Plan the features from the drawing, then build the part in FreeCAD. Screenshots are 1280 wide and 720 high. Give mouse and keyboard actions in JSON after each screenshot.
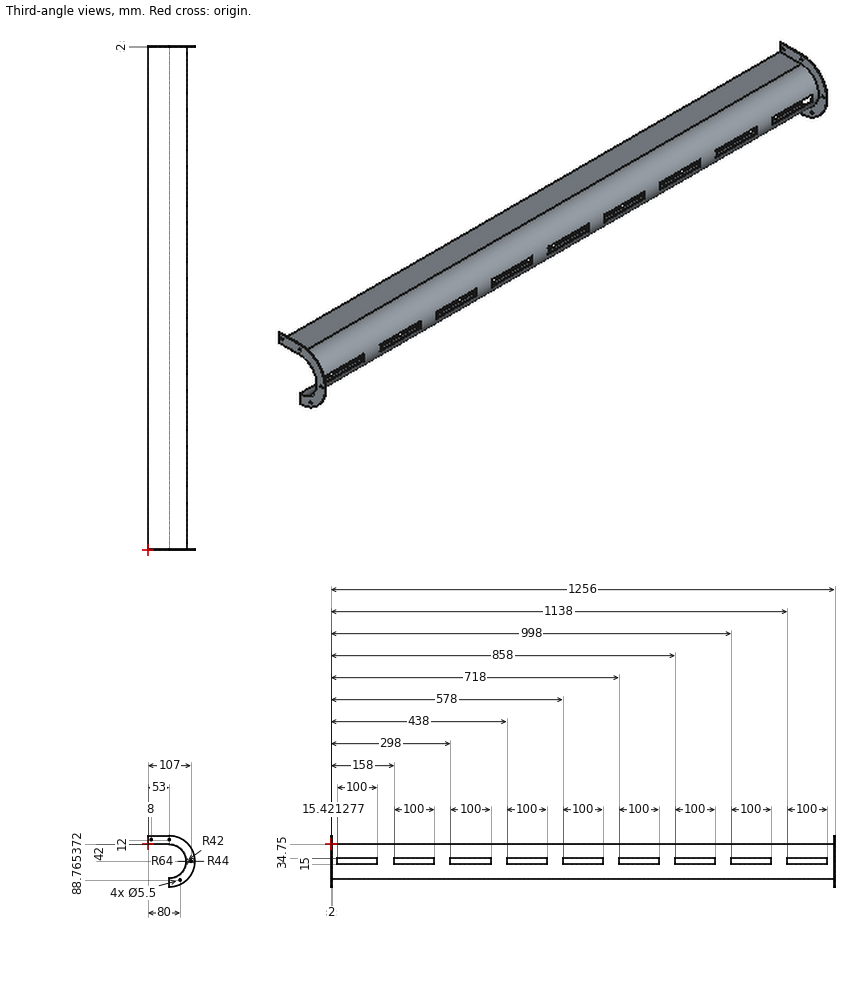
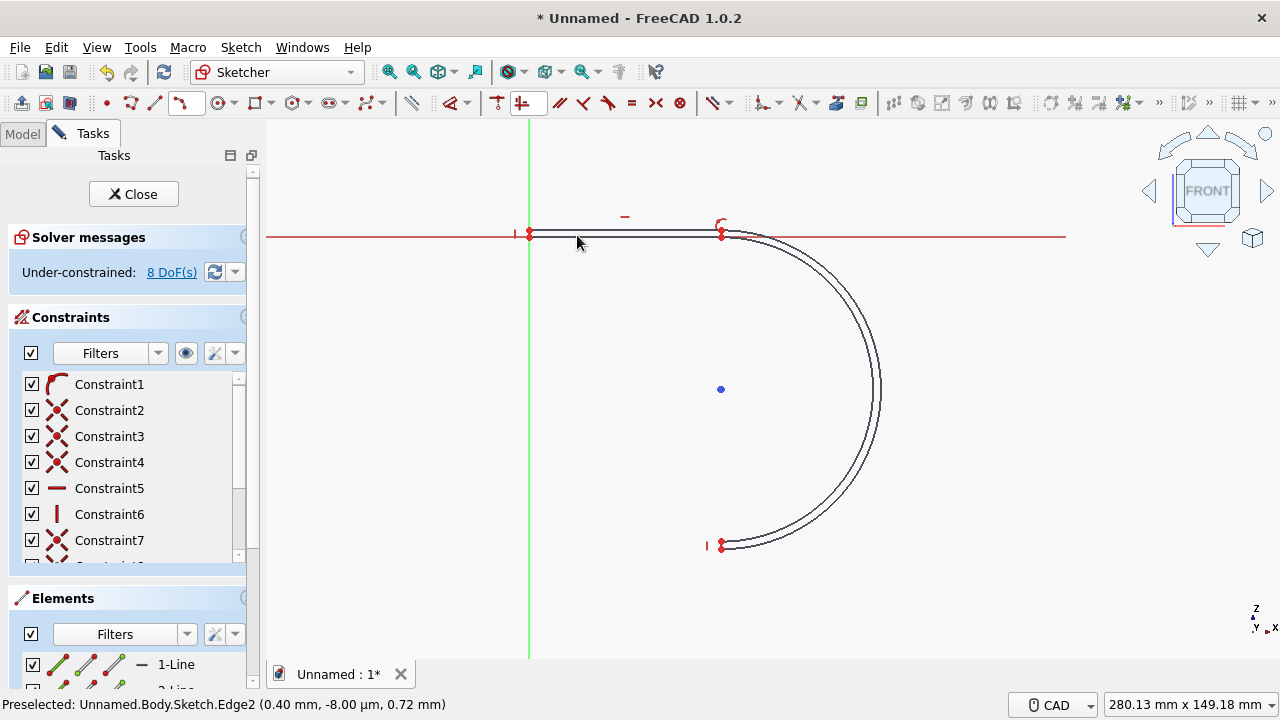
{"action": "scroll", "coordinate": [851, 483], "scroll_direction": "up", "scroll_amount": 3}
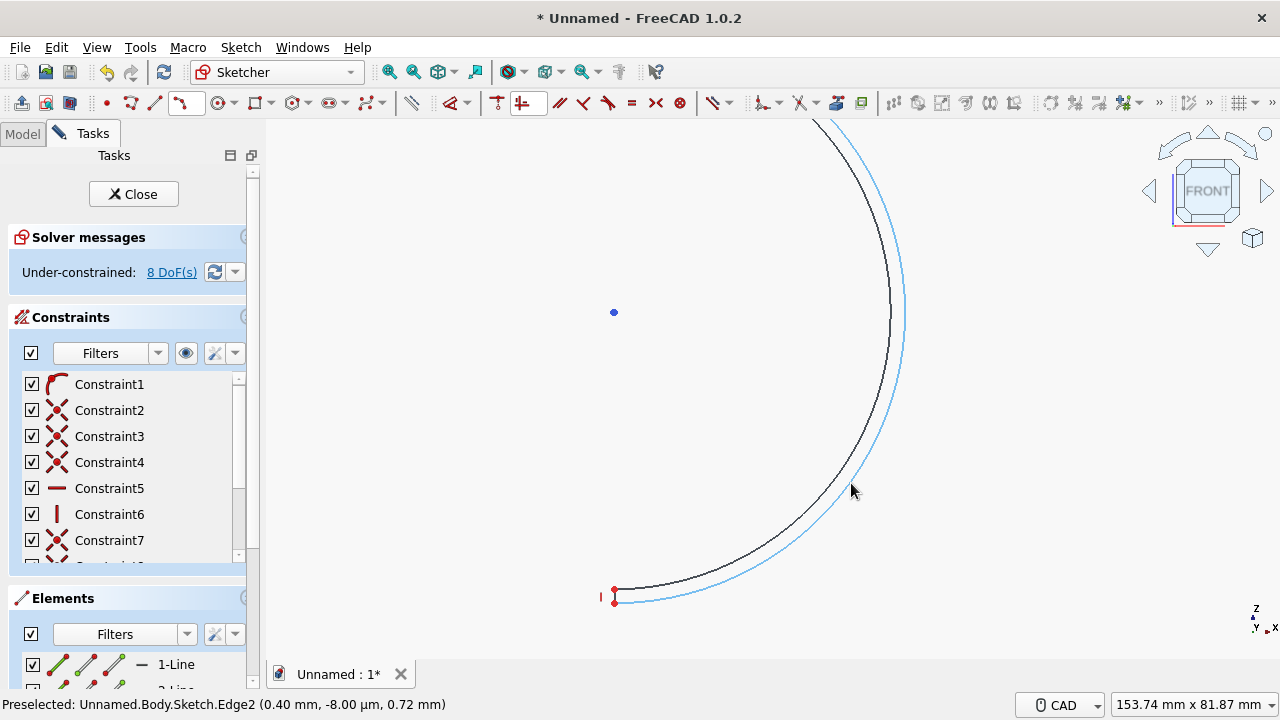
{"action": "left_click", "coordinate": [850, 483]}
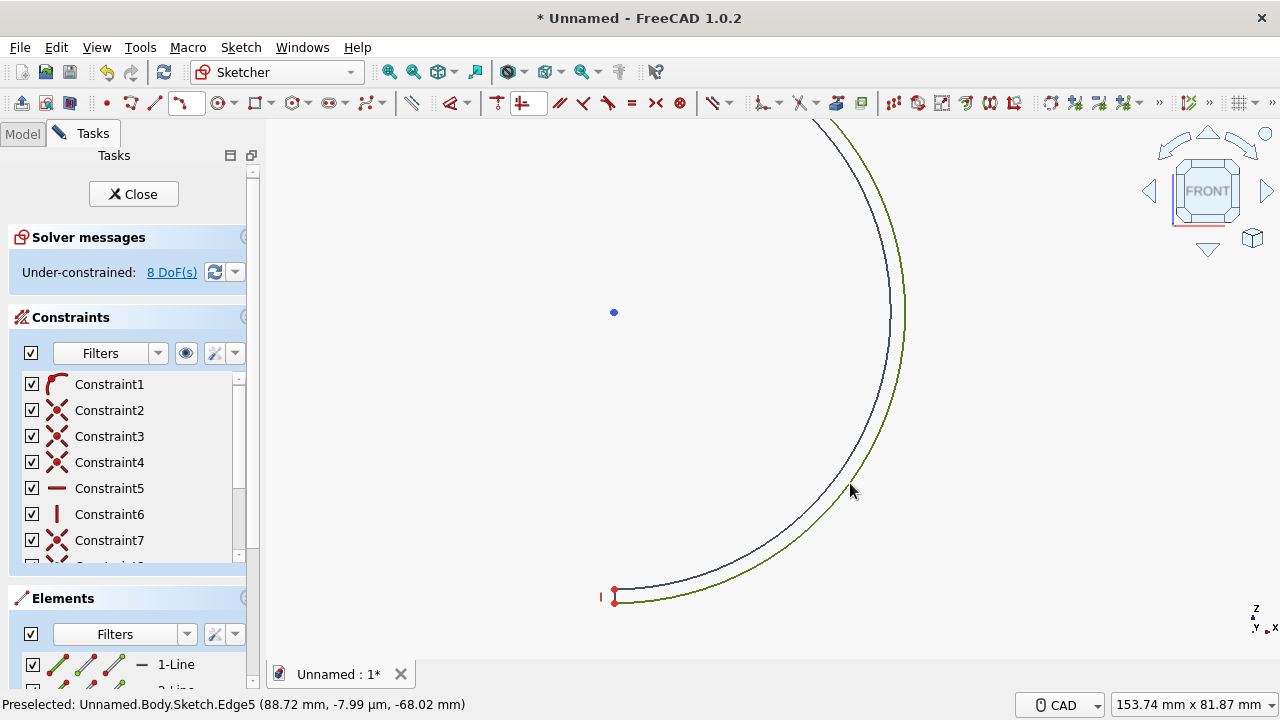
{"action": "left_click", "coordinate": [838, 475]}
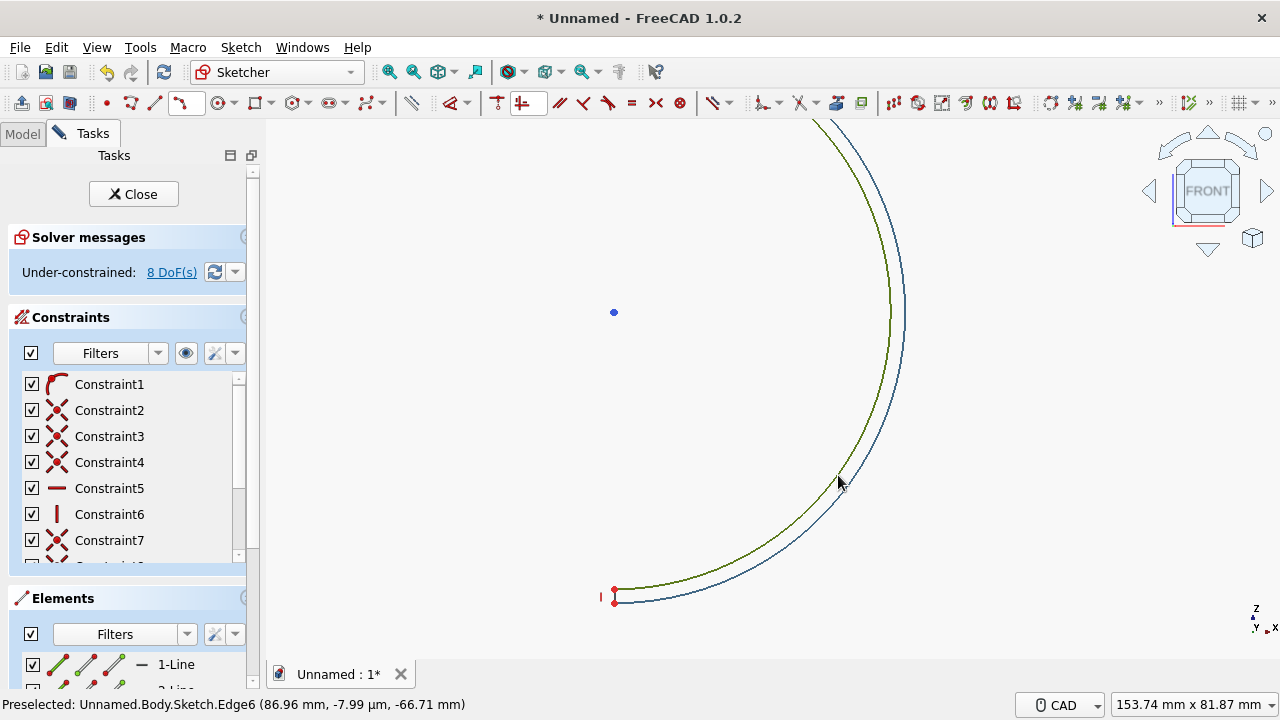
{"action": "key", "text": "c"}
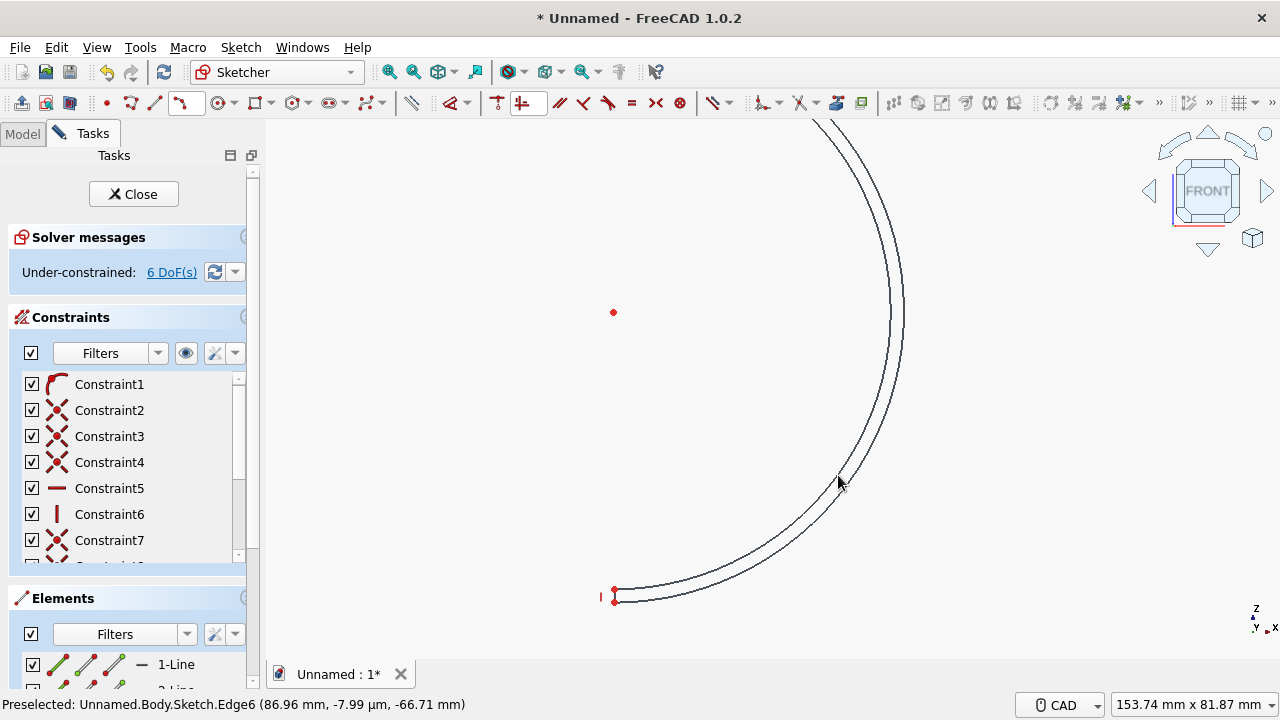
{"action": "left_click", "coordinate": [450, 104]}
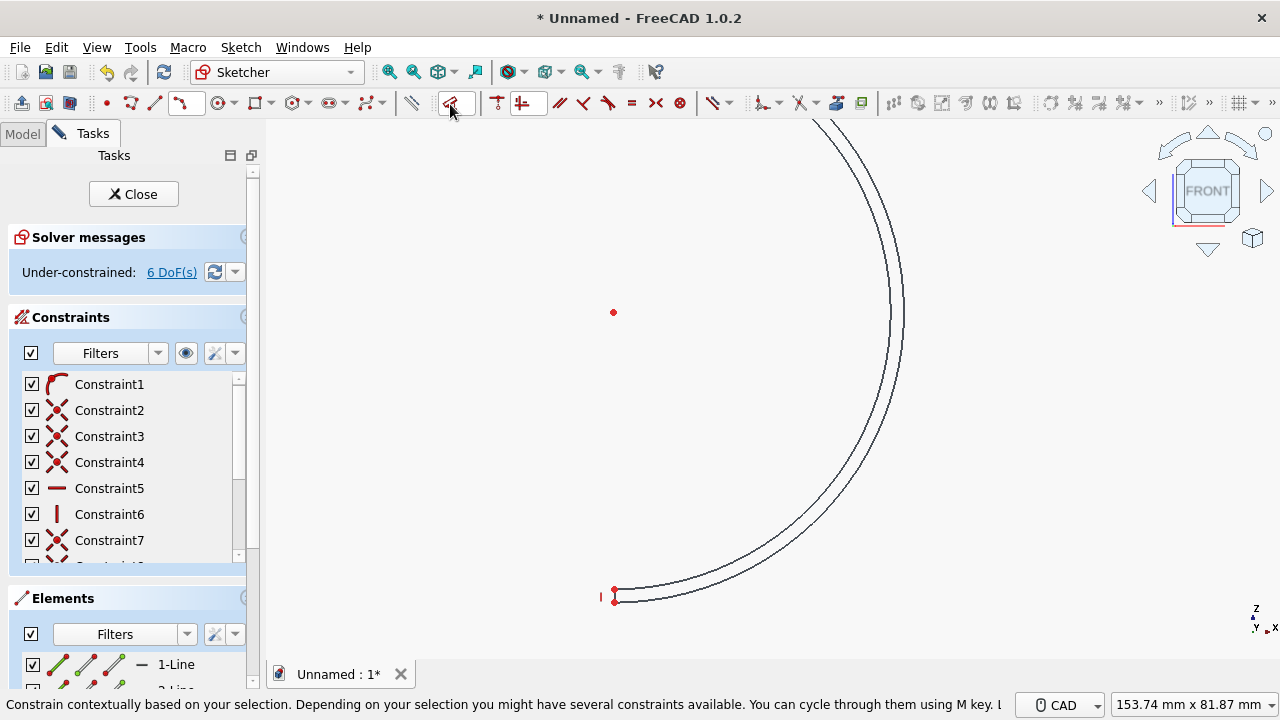
{"action": "left_click", "coordinate": [849, 482]}
{"action": "left_click", "coordinate": [875, 501]}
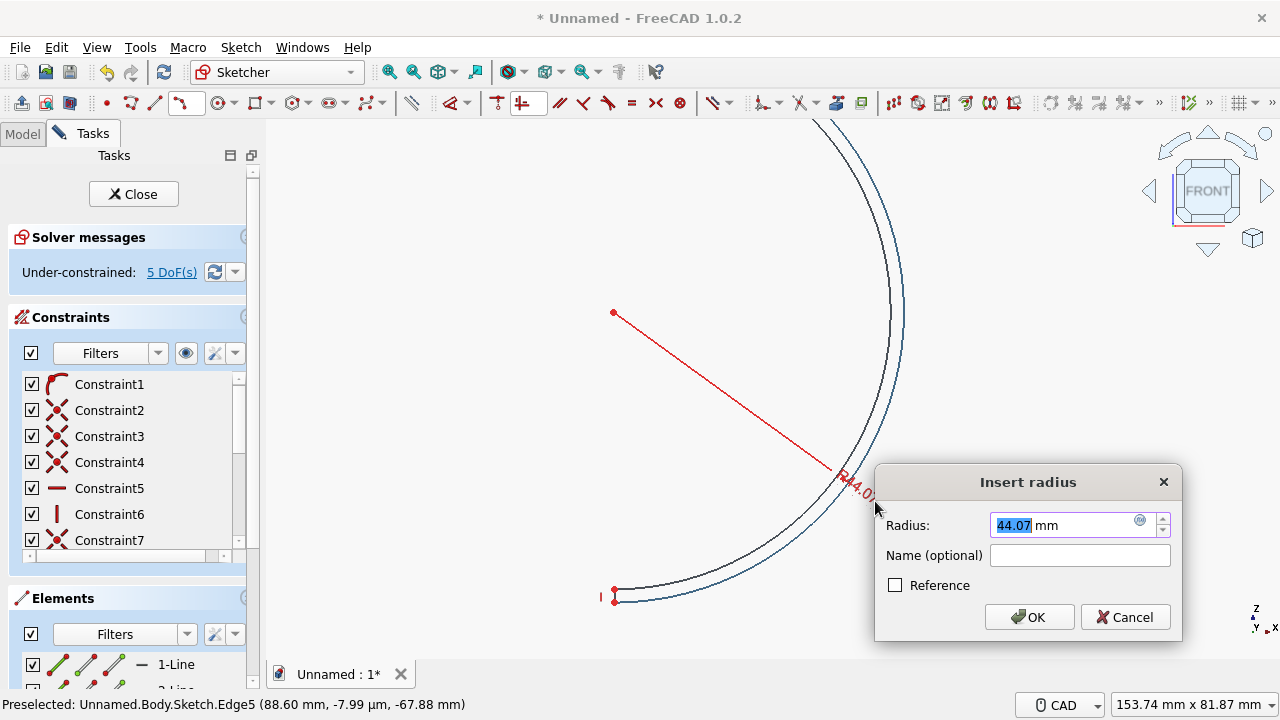
{"action": "type", "text": "44"}
{"action": "key", "text": "Return"}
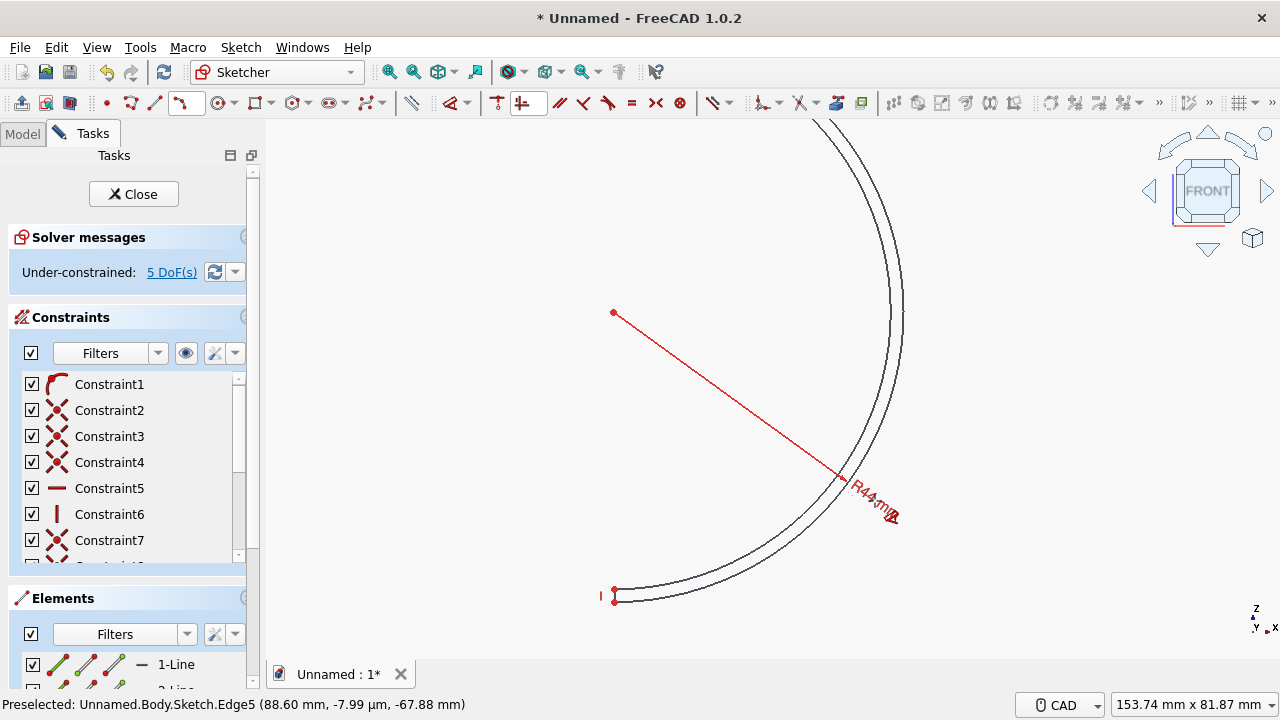
{"action": "left_click", "coordinate": [838, 475]}
{"action": "left_click", "coordinate": [746, 592]}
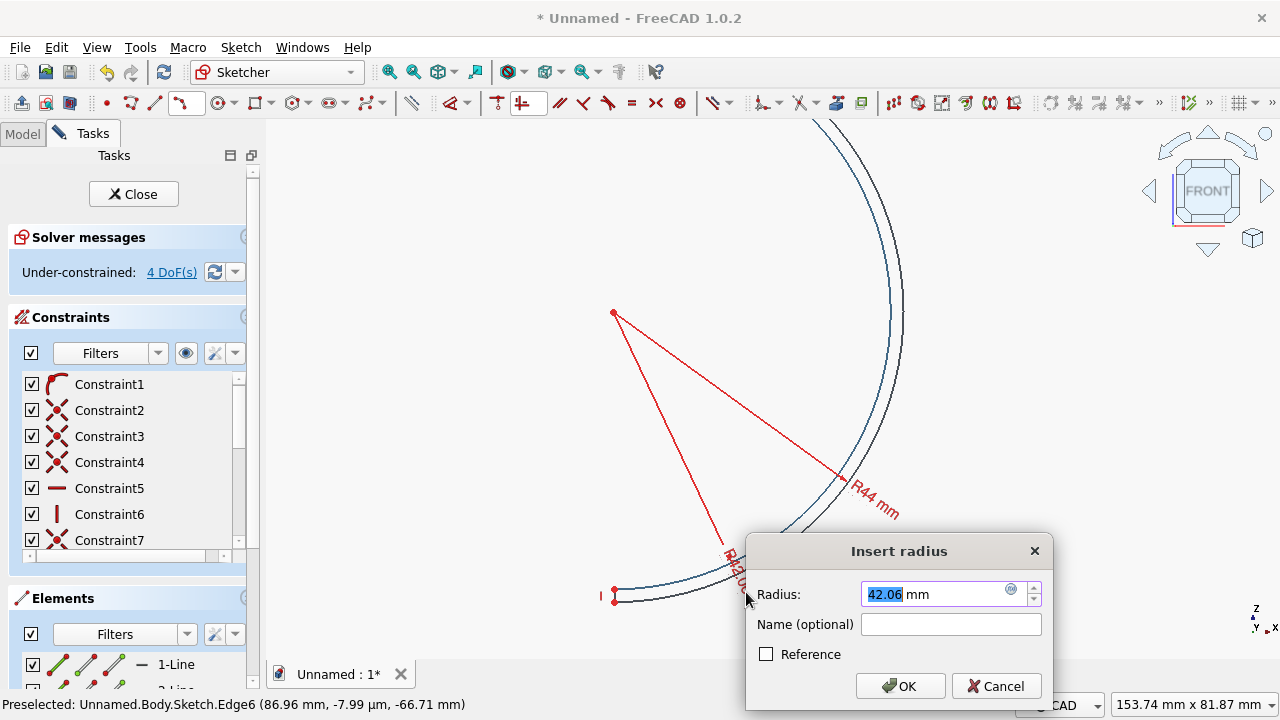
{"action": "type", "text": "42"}
{"action": "key", "text": "Return"}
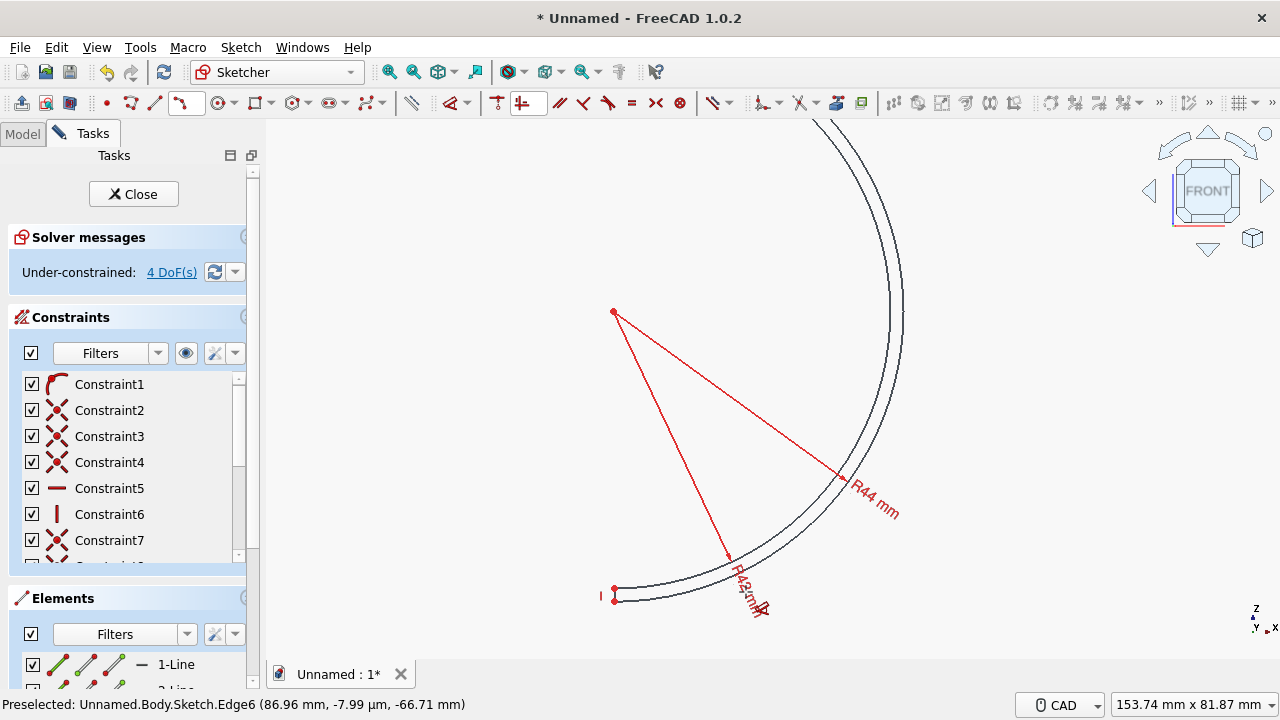
{"action": "scroll", "coordinate": [851, 483], "scroll_direction": "down", "scroll_amount": 3}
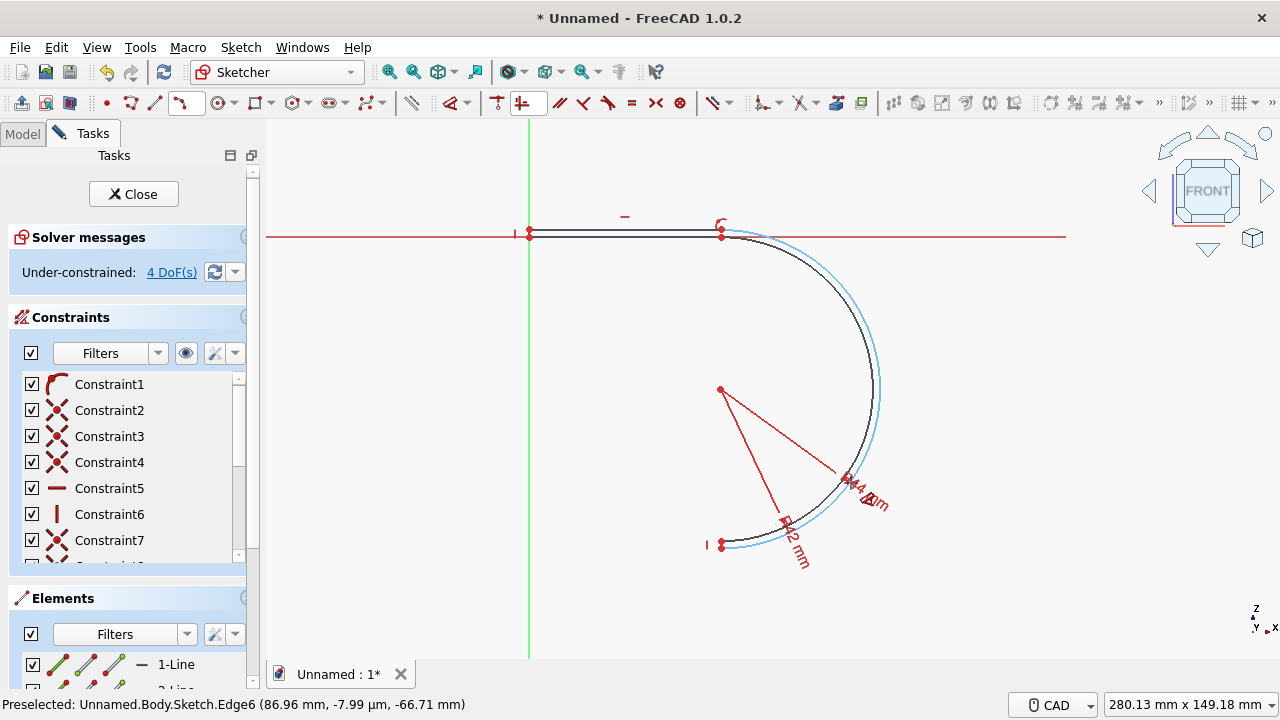
{"action": "scroll", "coordinate": [664, 237], "scroll_direction": "up", "scroll_amount": 4}